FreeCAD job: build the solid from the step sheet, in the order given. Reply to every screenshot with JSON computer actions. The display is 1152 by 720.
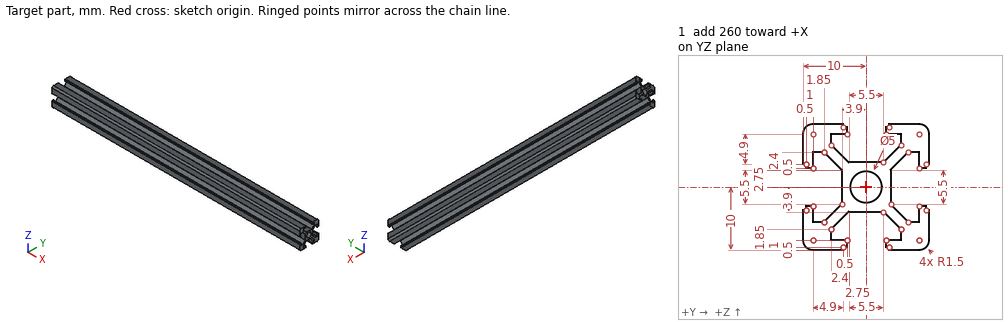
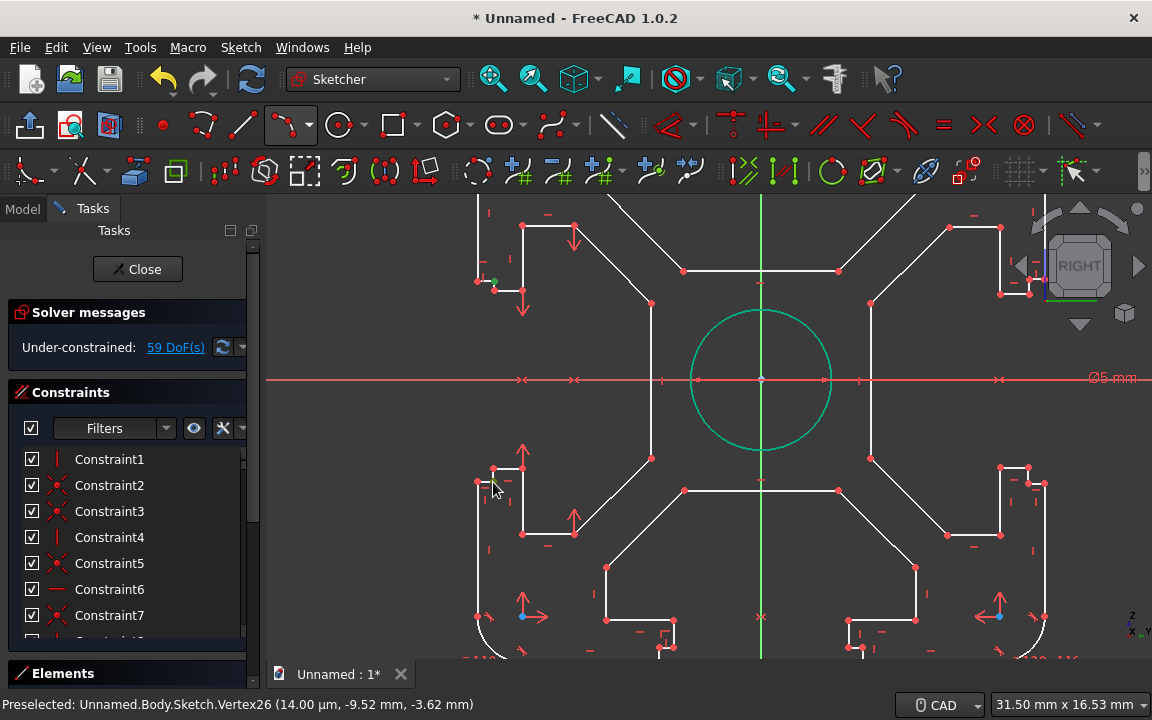
{"action": "left_click", "coordinate": [344, 380]}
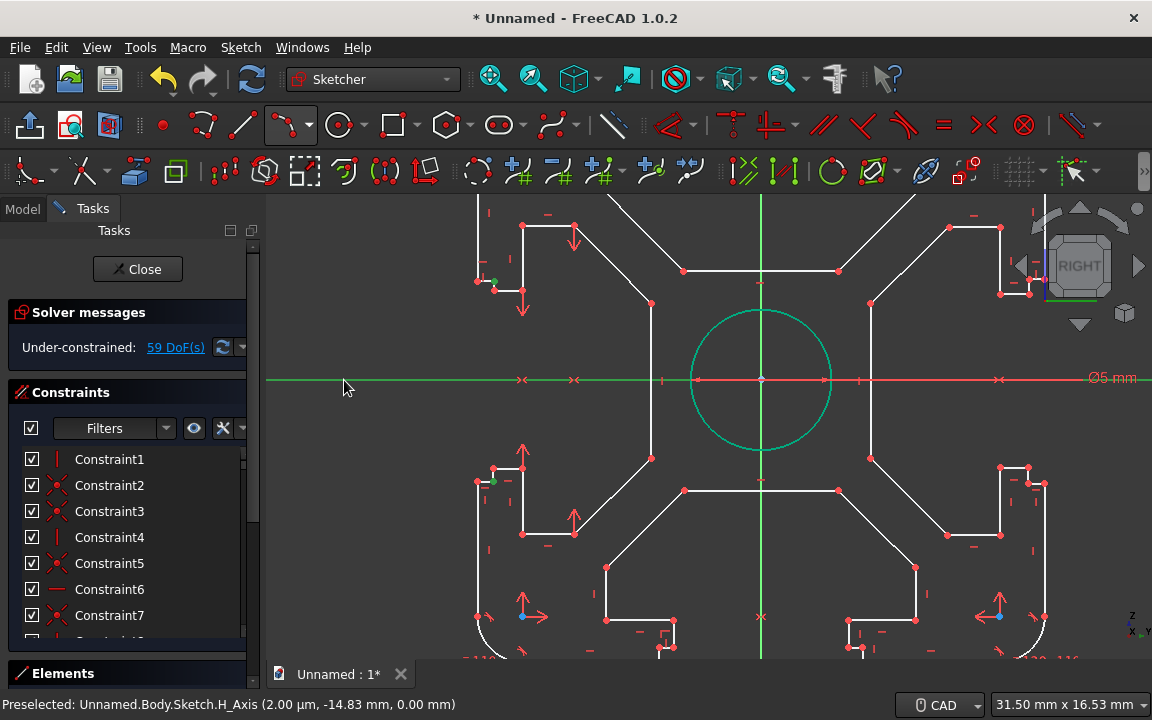
{"action": "key", "text": "s"}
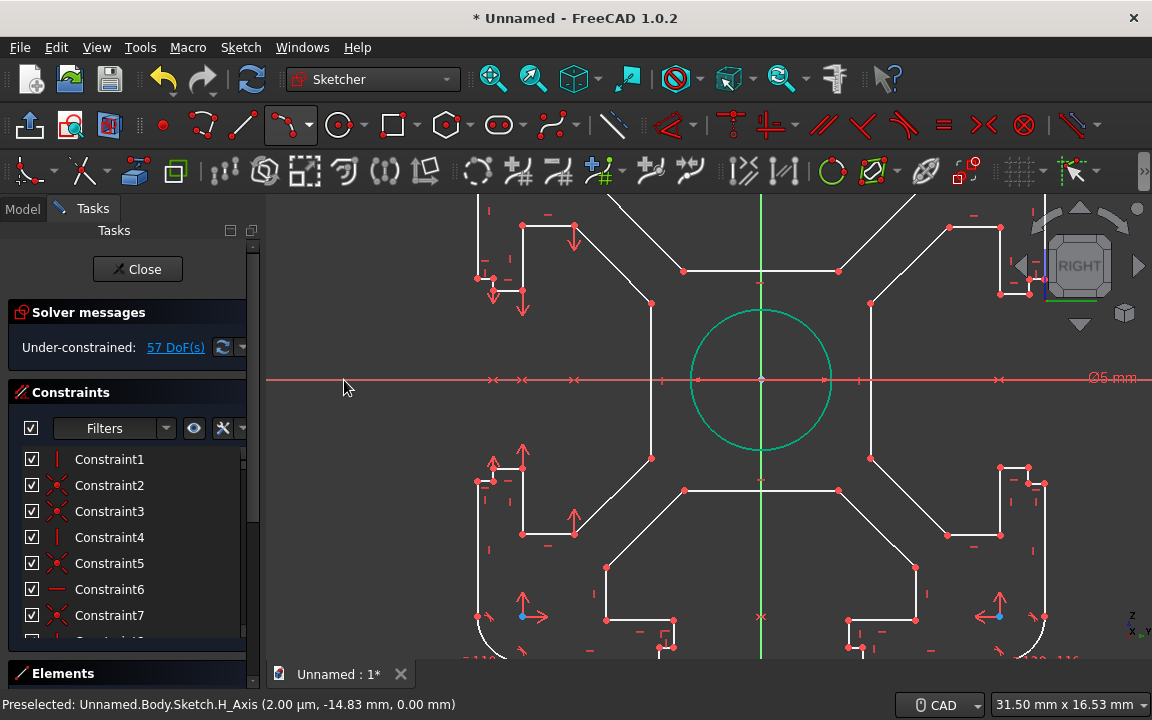
{"action": "left_click", "coordinate": [606, 568]}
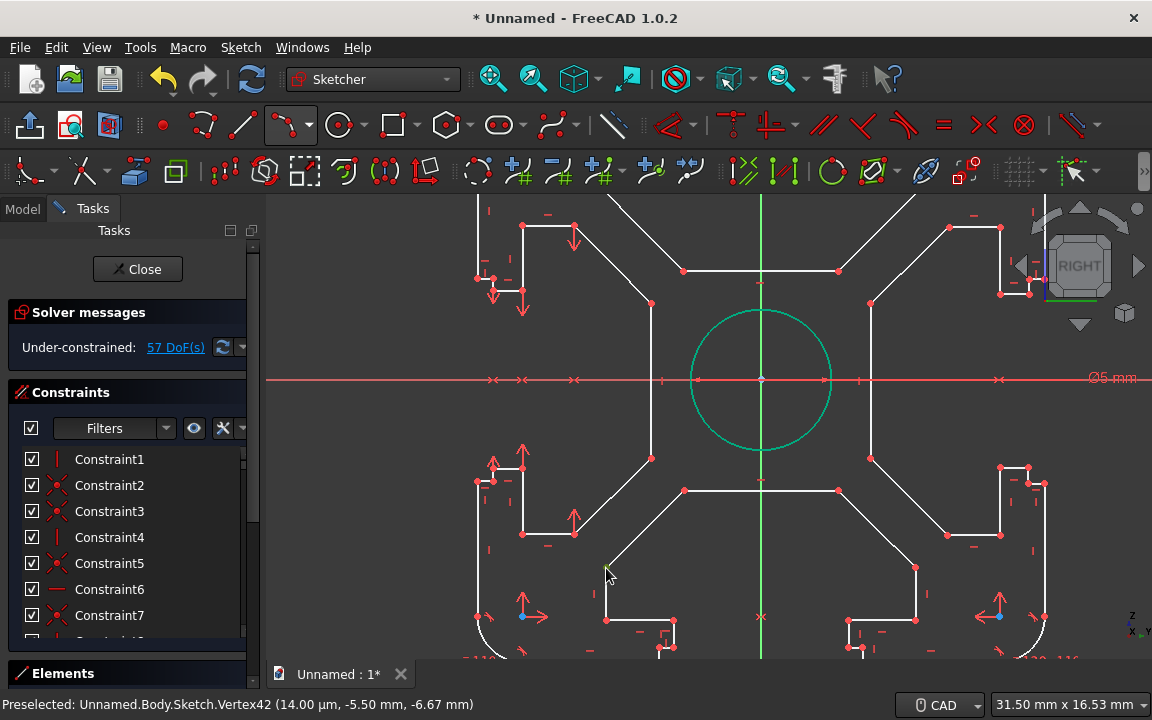
{"action": "left_click", "coordinate": [916, 568]}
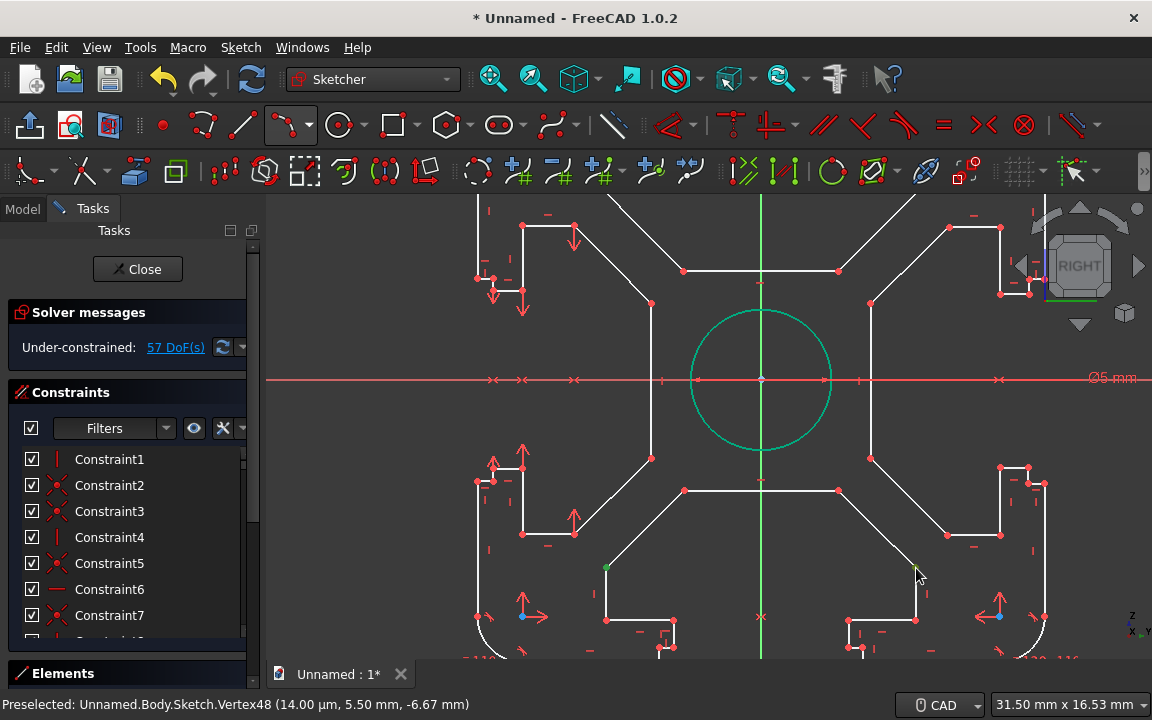
{"action": "left_click", "coordinate": [761, 602]}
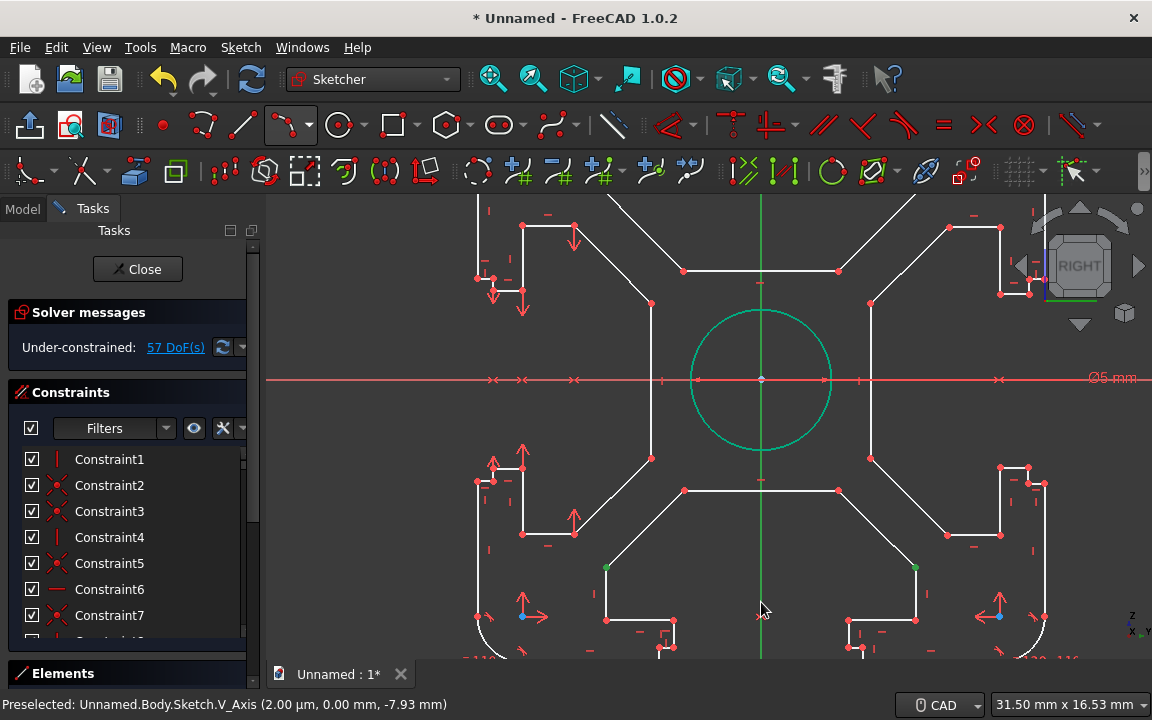
{"action": "key", "text": "s"}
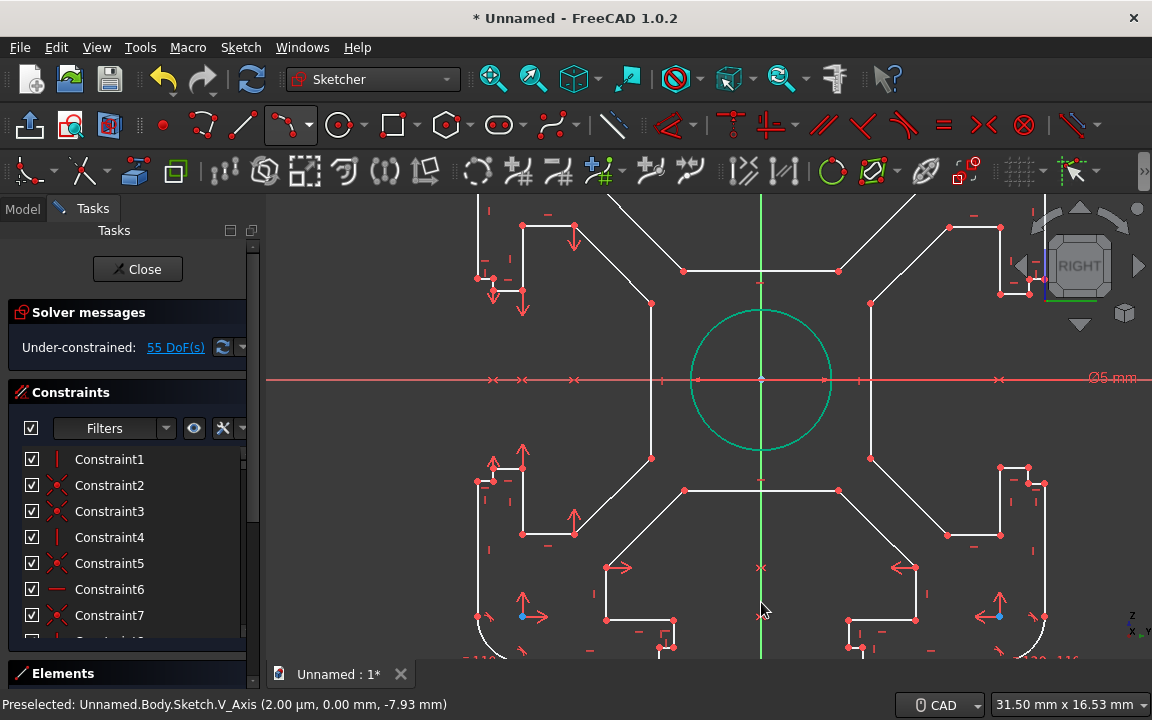
{"action": "left_click", "coordinate": [674, 620]}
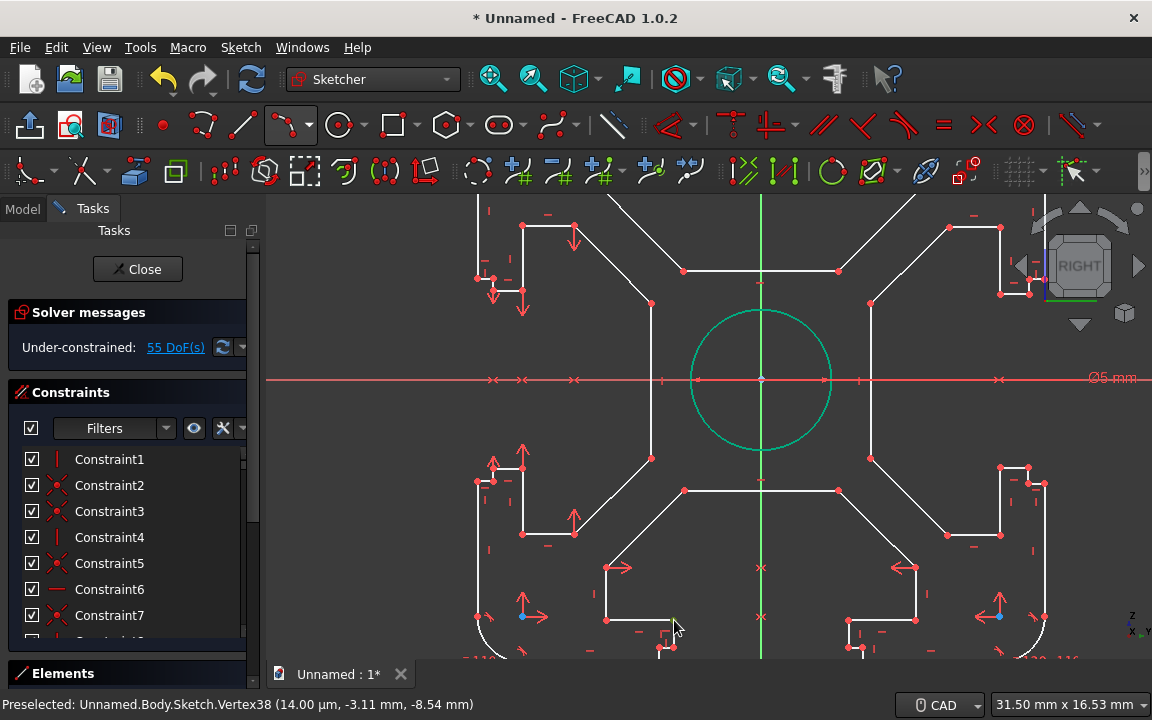
{"action": "left_click", "coordinate": [849, 620]}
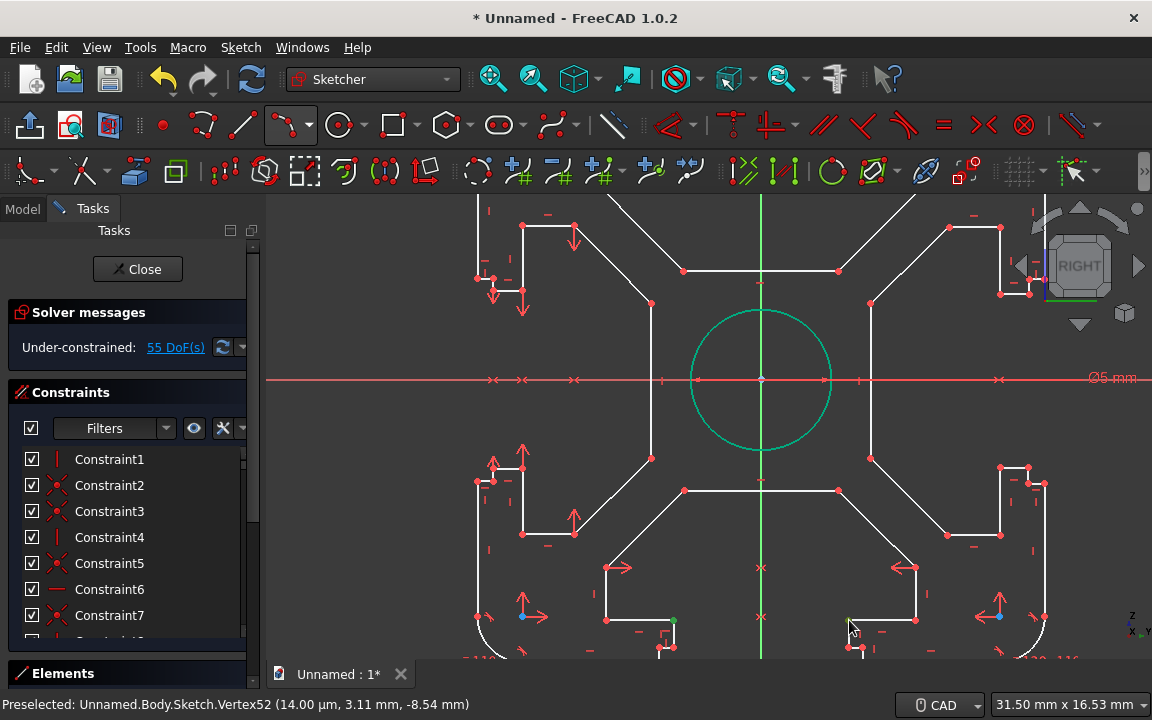
{"action": "left_click", "coordinate": [761, 602]}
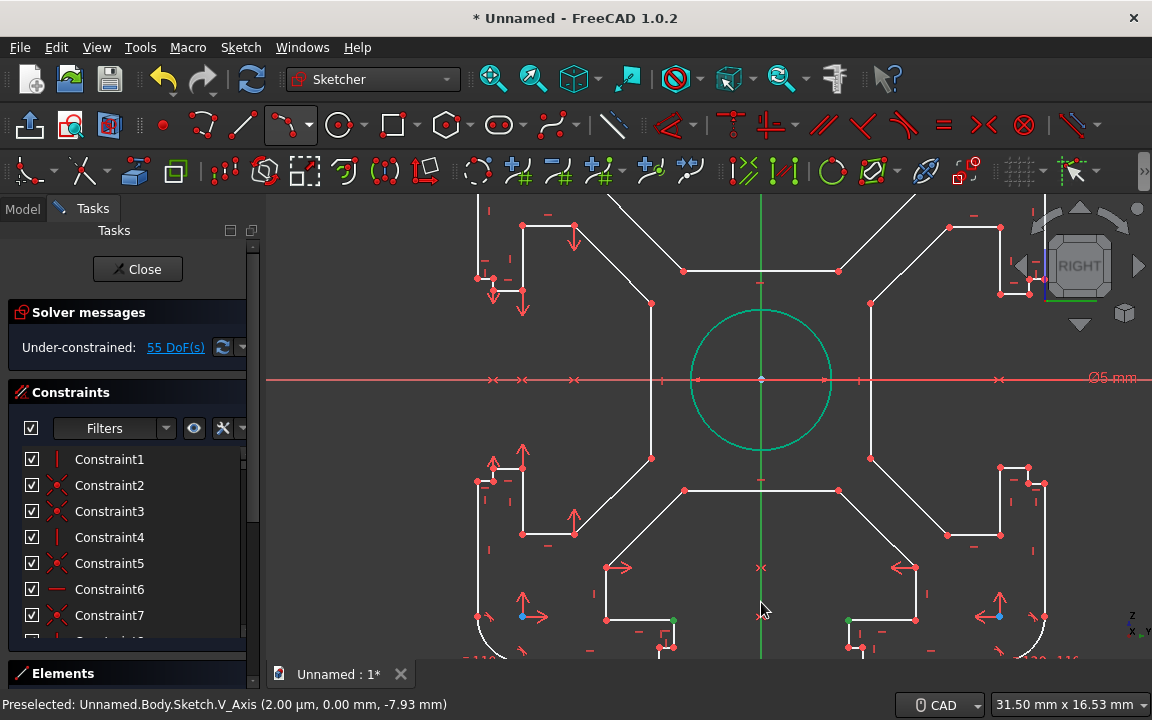
{"action": "key", "text": "s"}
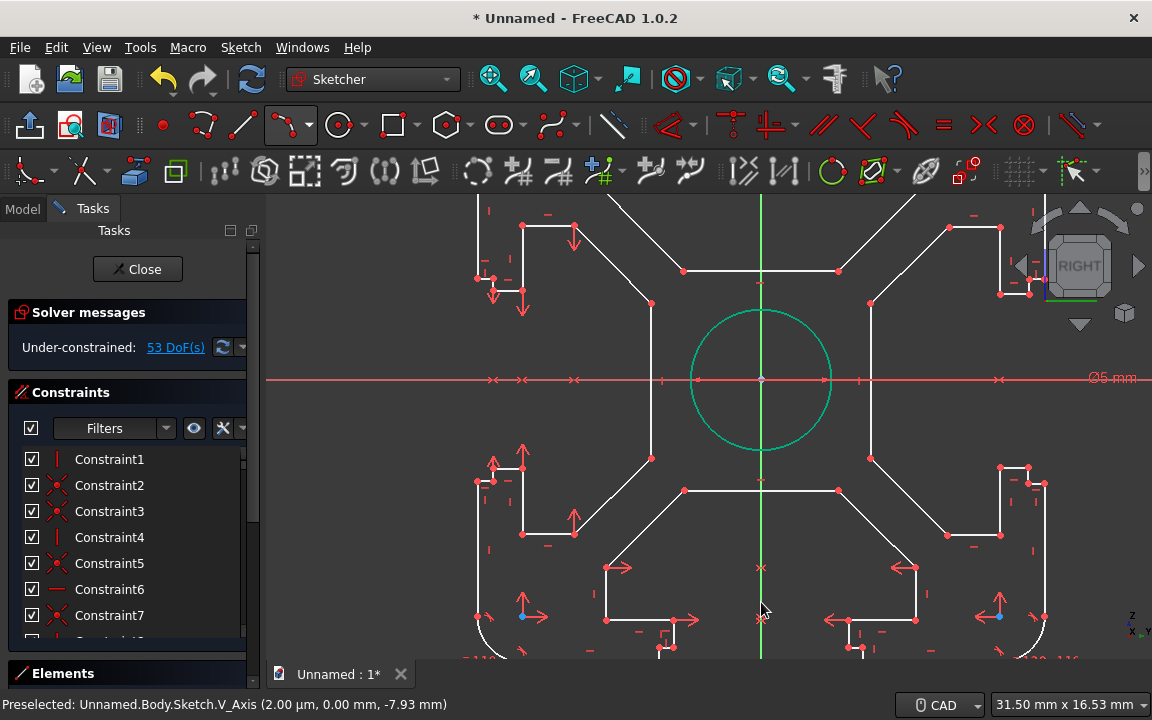
{"action": "scroll", "coordinate": [494, 483], "scroll_direction": "down", "scroll_amount": 3}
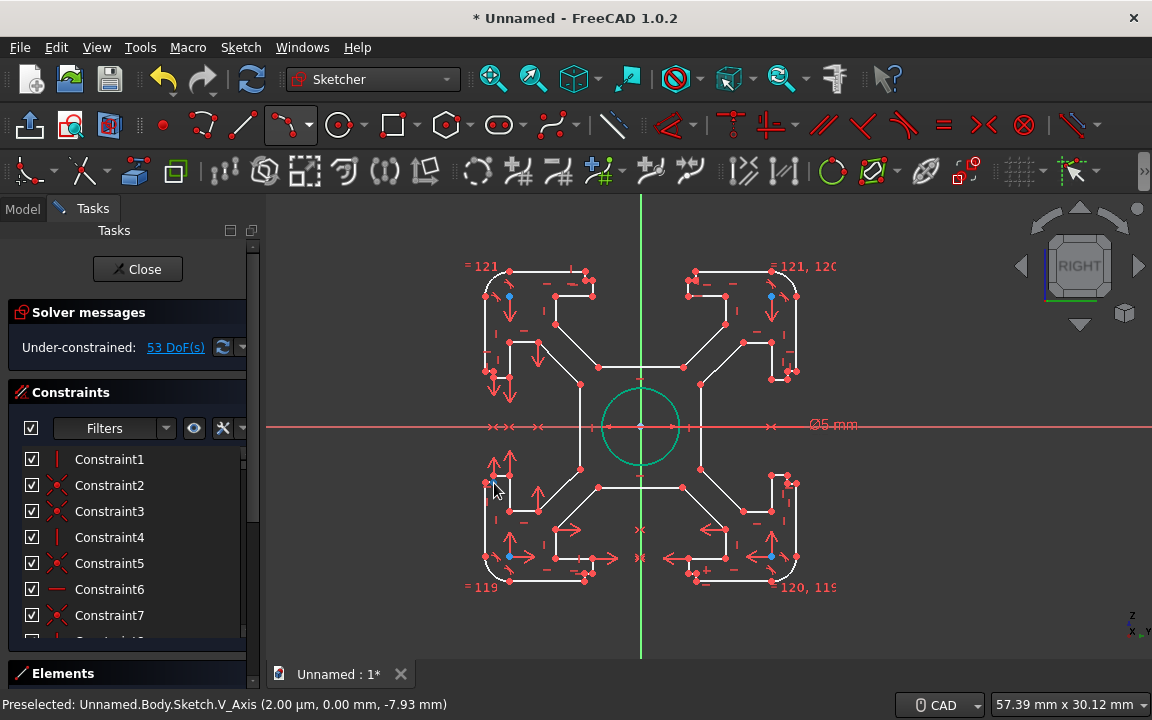
{"action": "scroll", "coordinate": [585, 574], "scroll_direction": "up", "scroll_amount": 3}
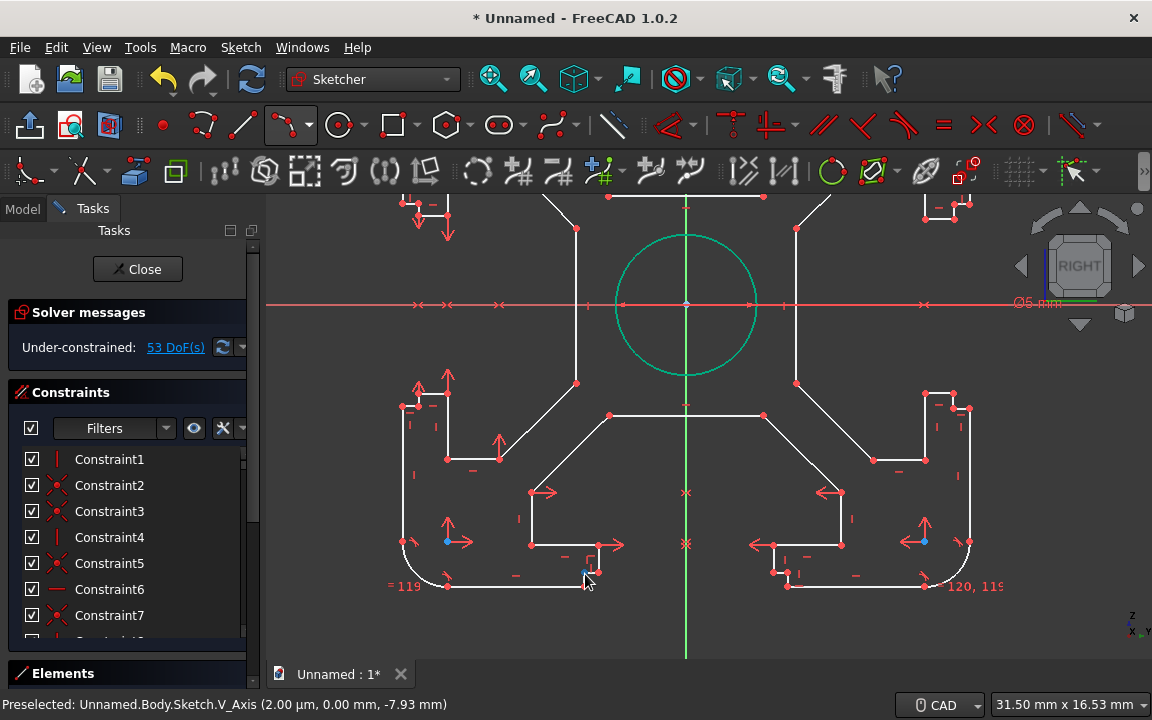
{"action": "left_click", "coordinate": [584, 573]}